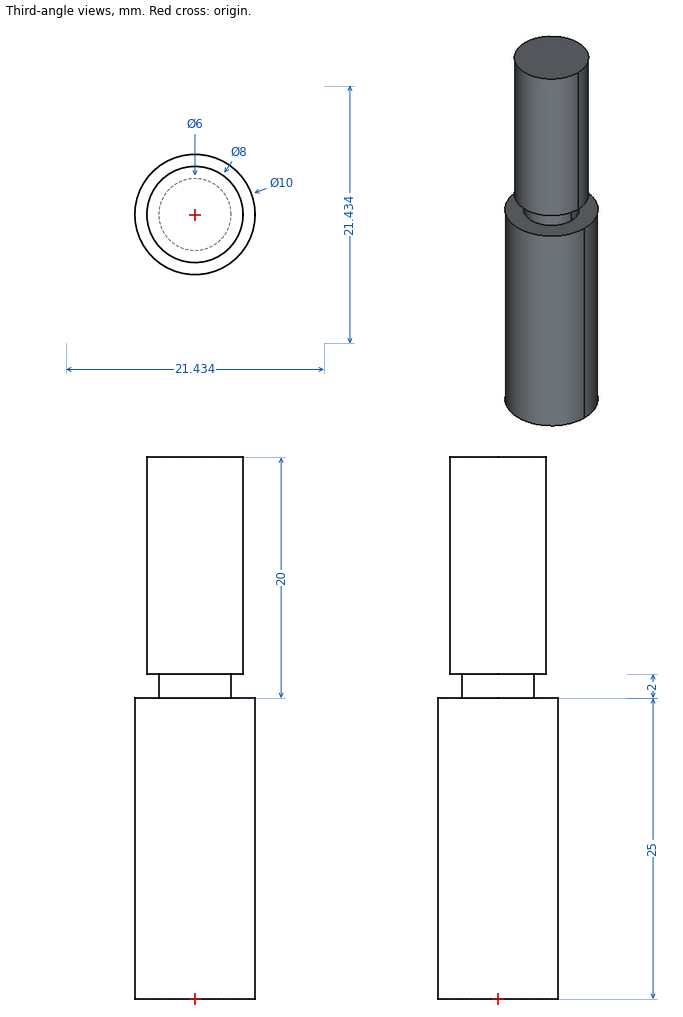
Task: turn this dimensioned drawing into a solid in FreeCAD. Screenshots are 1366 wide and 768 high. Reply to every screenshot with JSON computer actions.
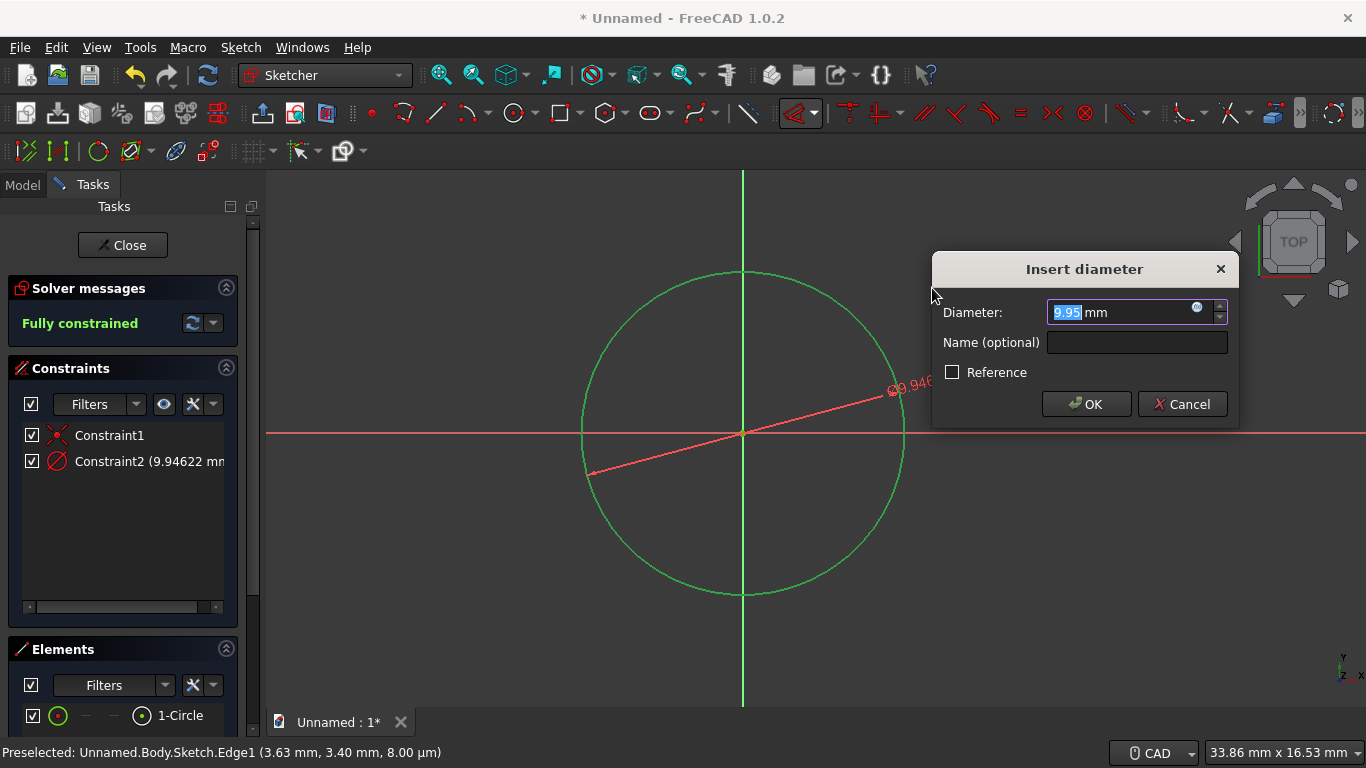
{"action": "type", "text": "10"}
{"action": "key", "text": "Return"}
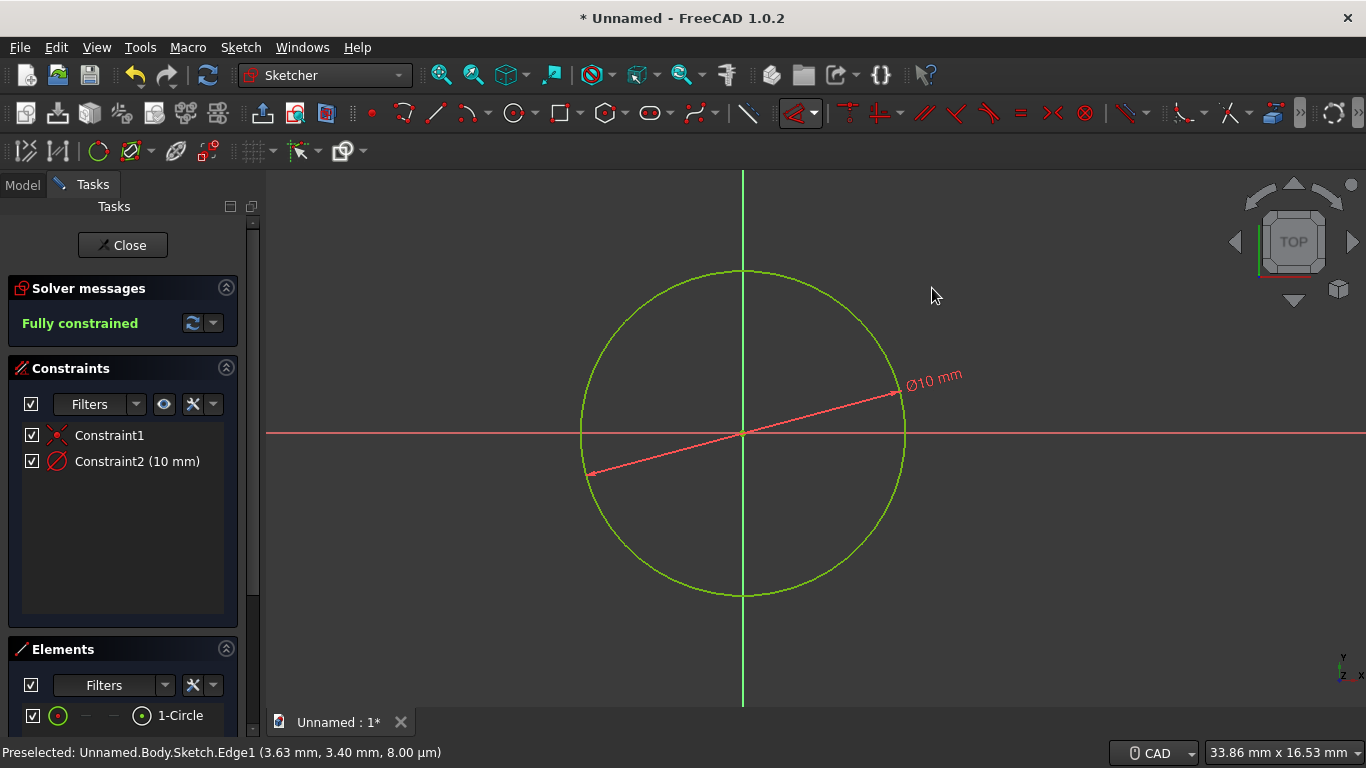
{"action": "left_click", "coordinate": [123, 245]}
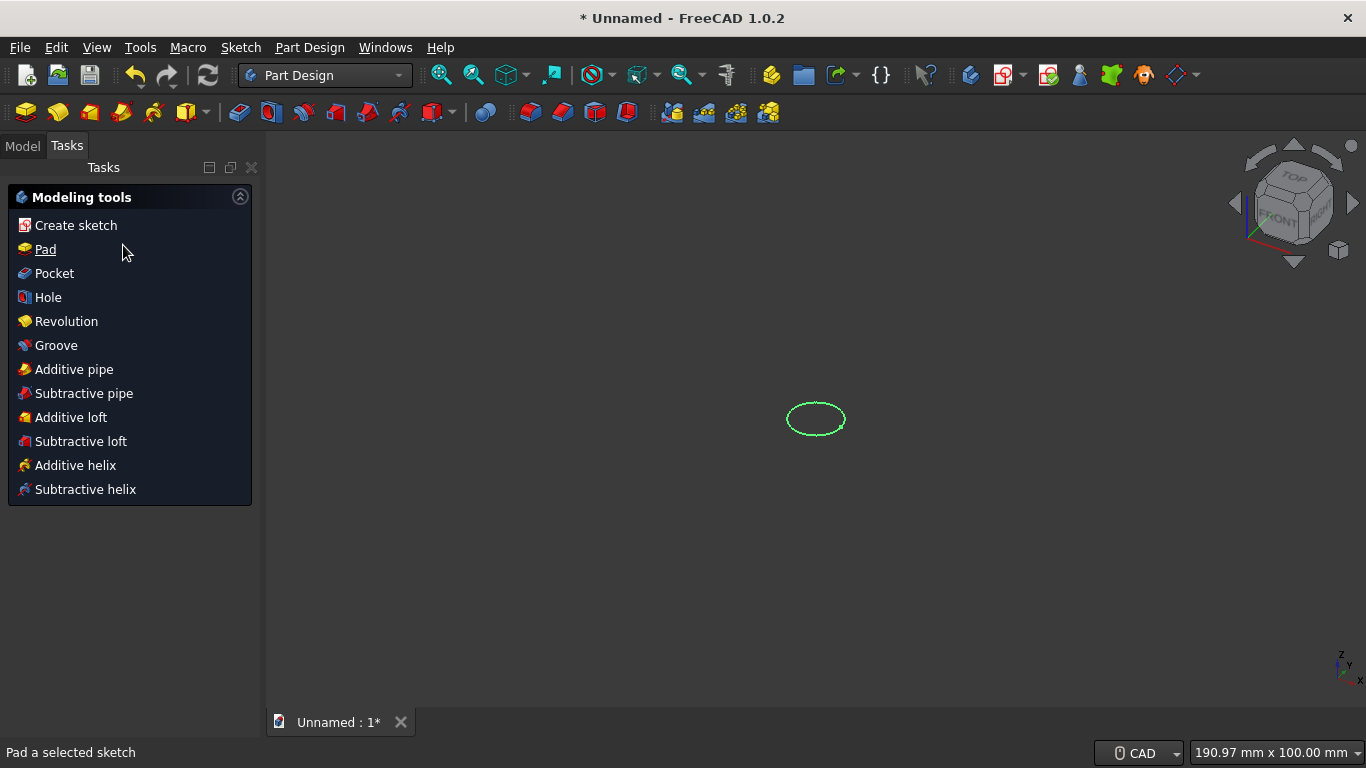
{"action": "left_click", "coordinate": [26, 112]}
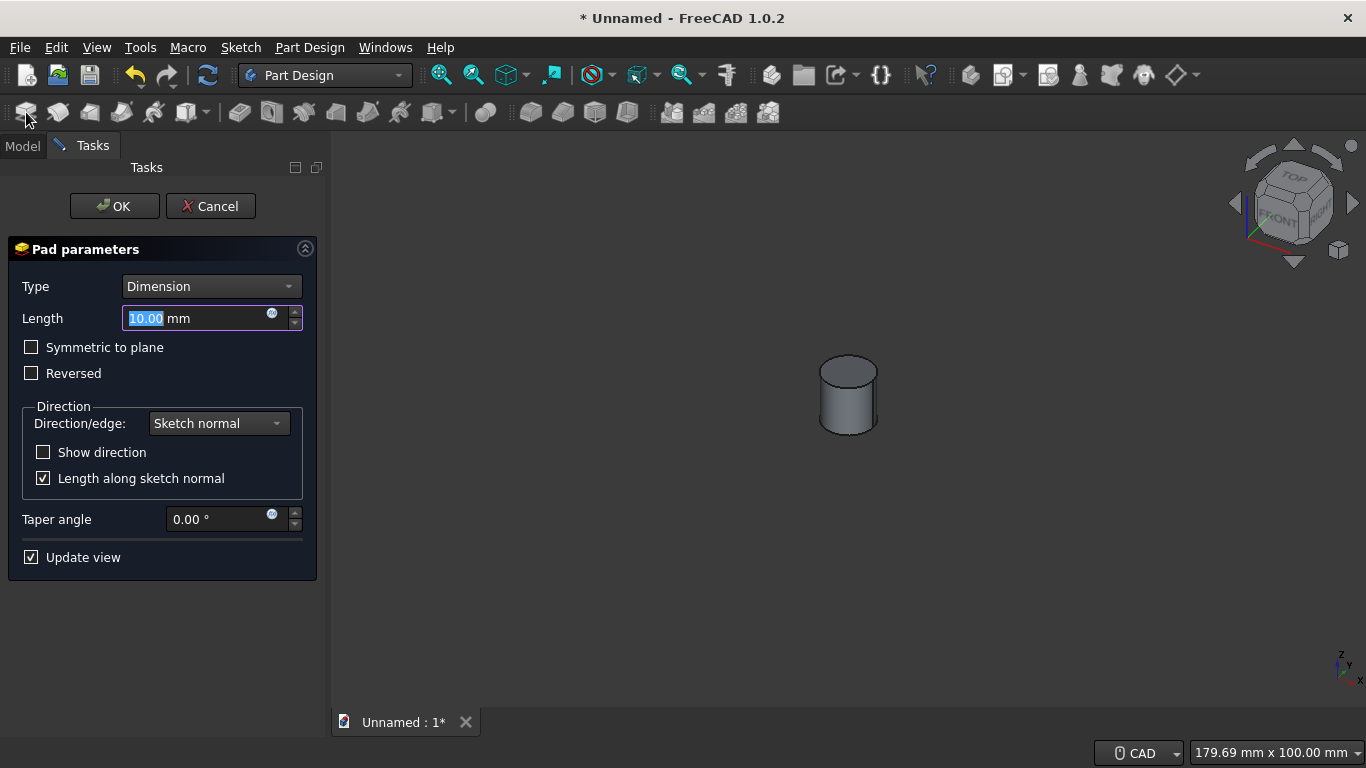
{"action": "type", "text": "25"}
{"action": "key", "text": "Tab"}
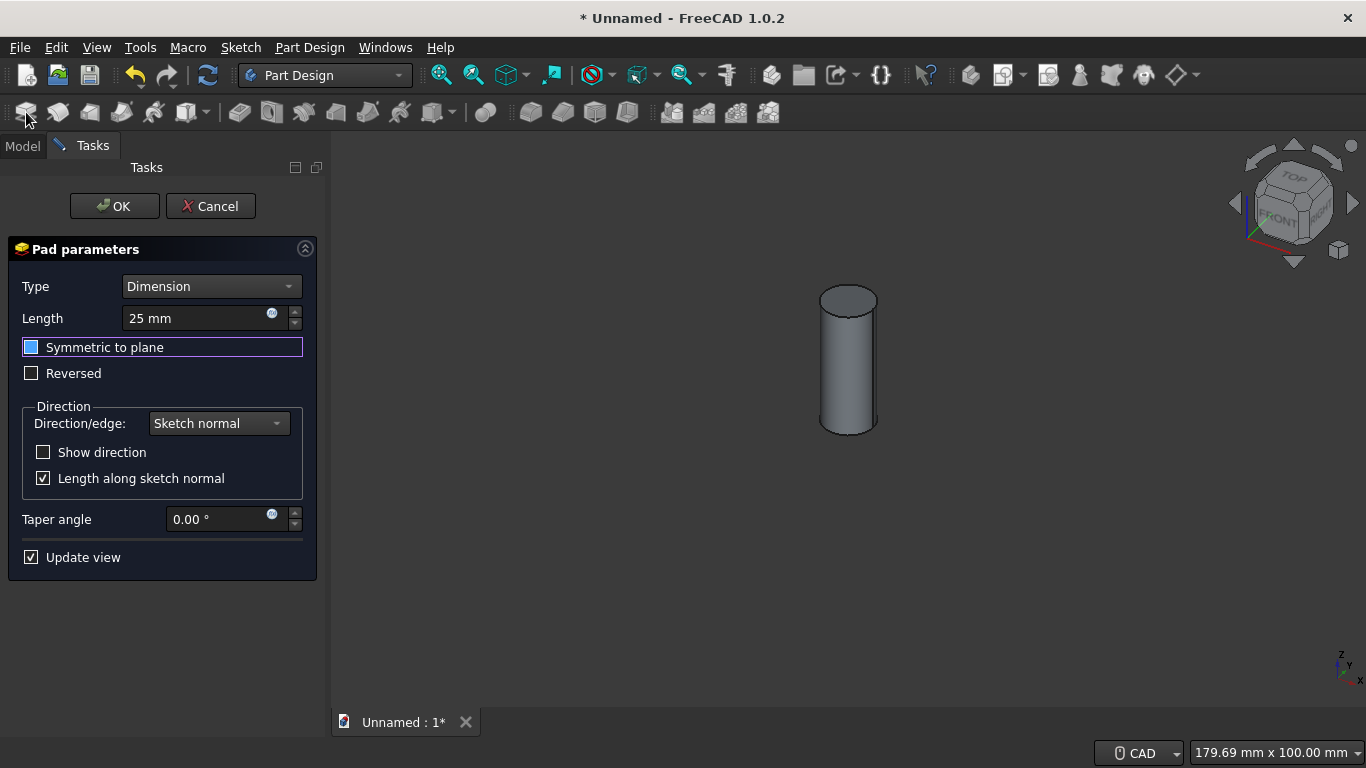
{"action": "left_click", "coordinate": [115, 206]}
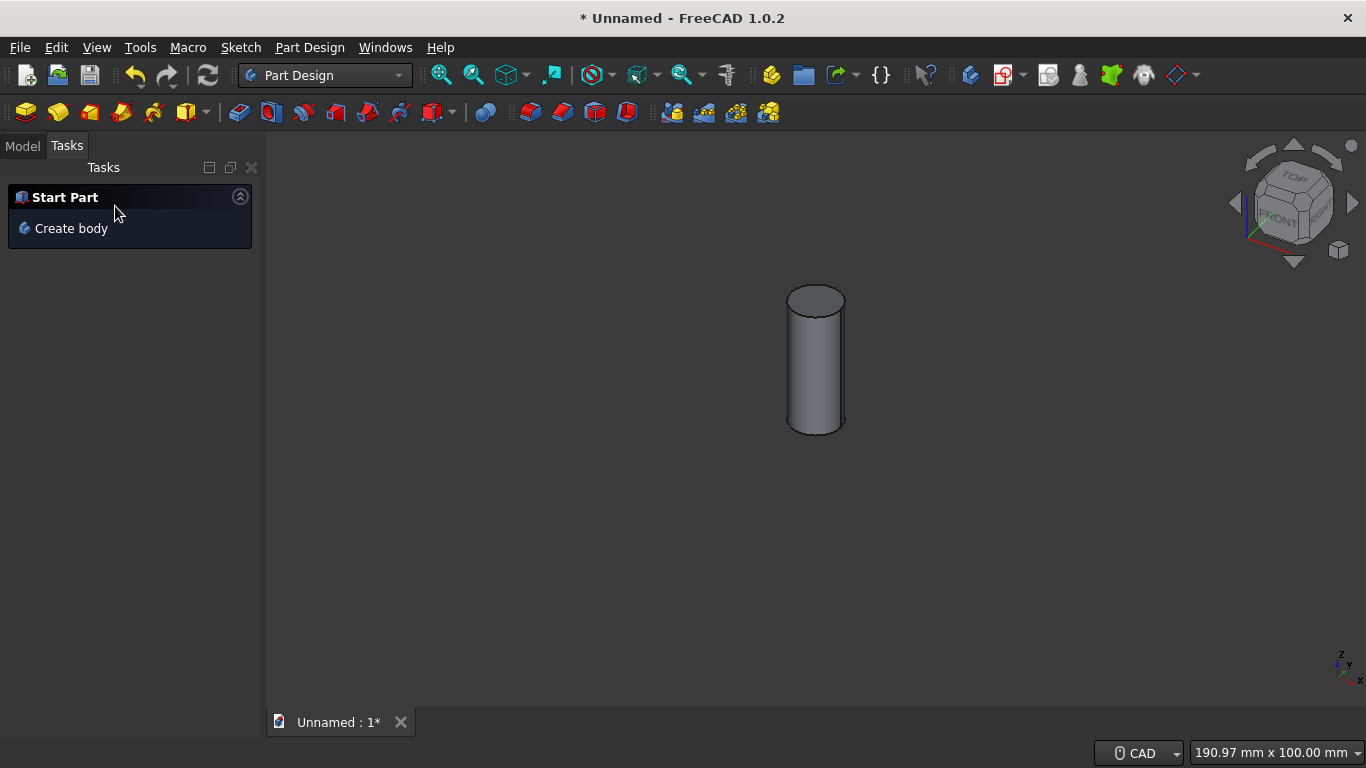
{"action": "left_click", "coordinate": [442, 76]}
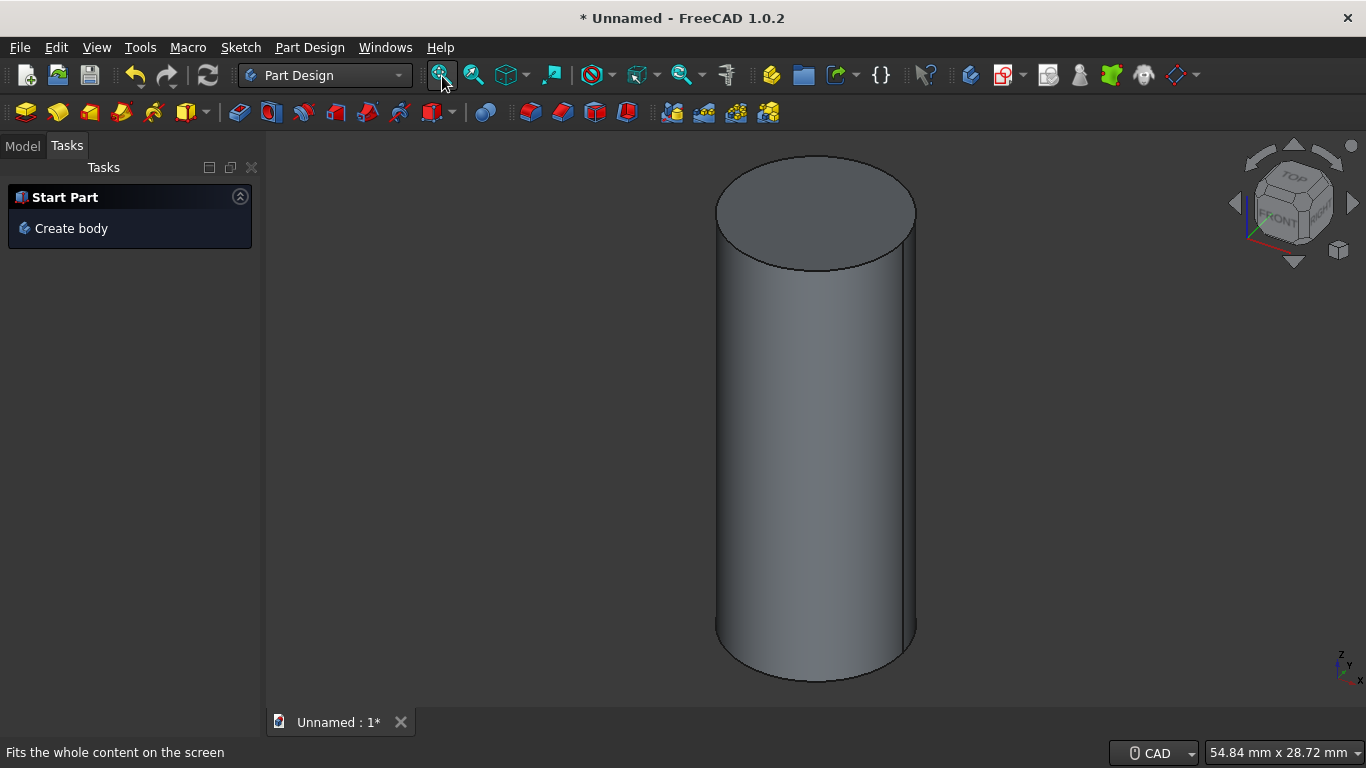
{"action": "left_click", "coordinate": [816, 213]}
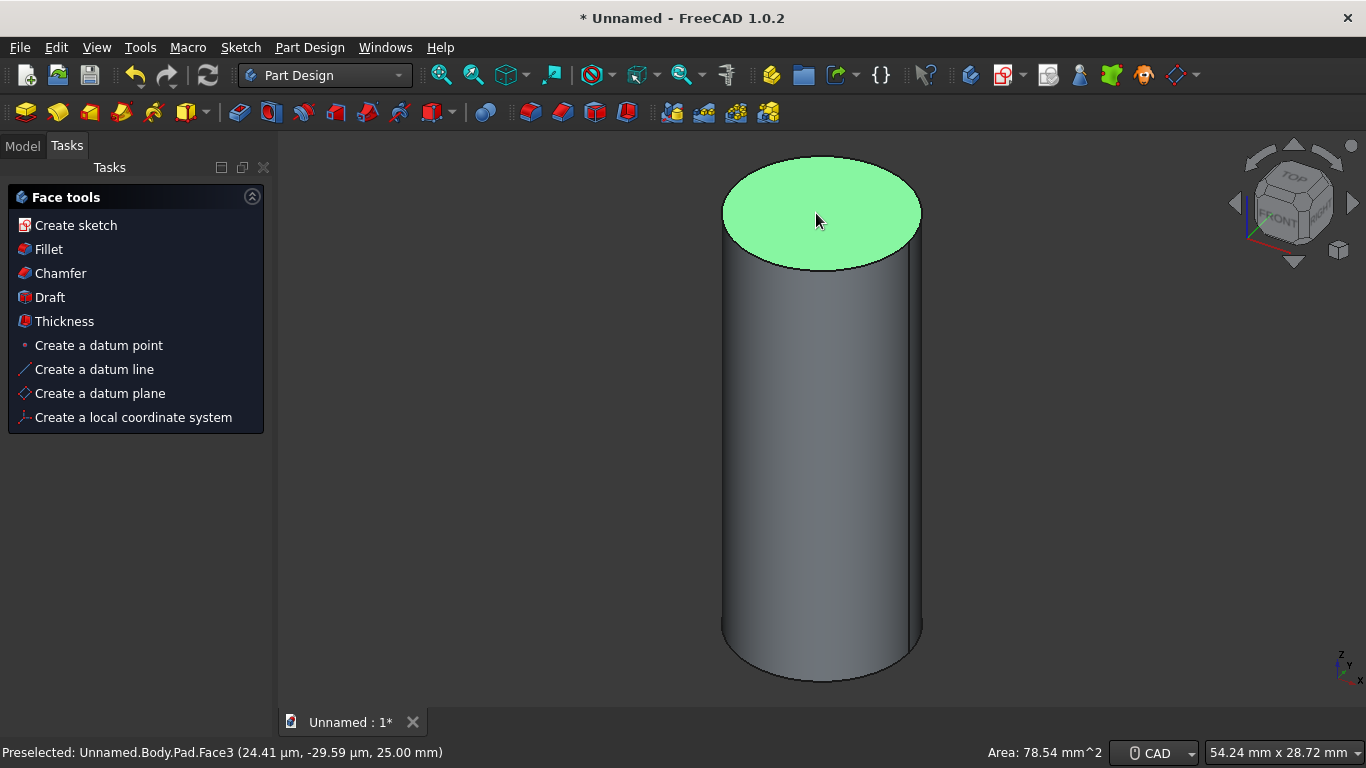
{"action": "left_click", "coordinate": [1004, 76]}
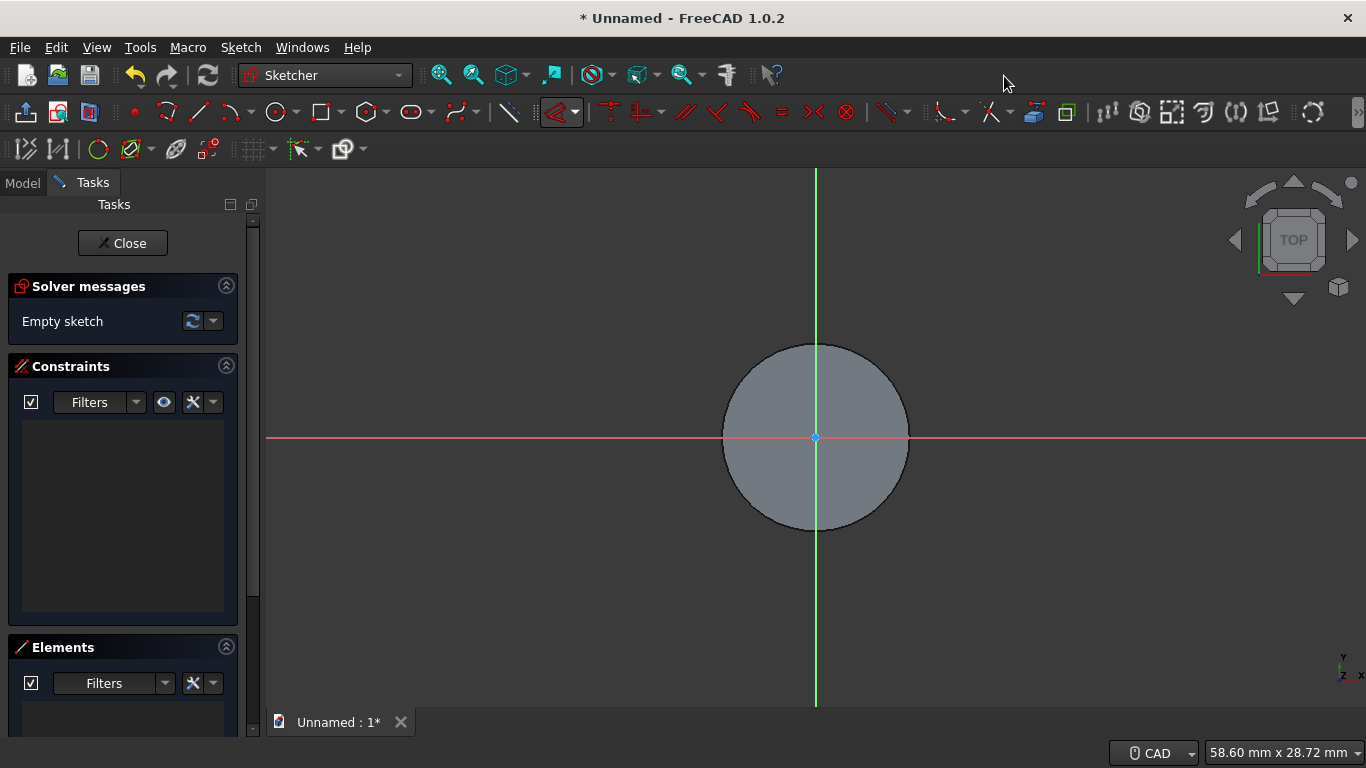
{"action": "scroll", "coordinate": [872, 438], "scroll_direction": "up", "scroll_amount": 4}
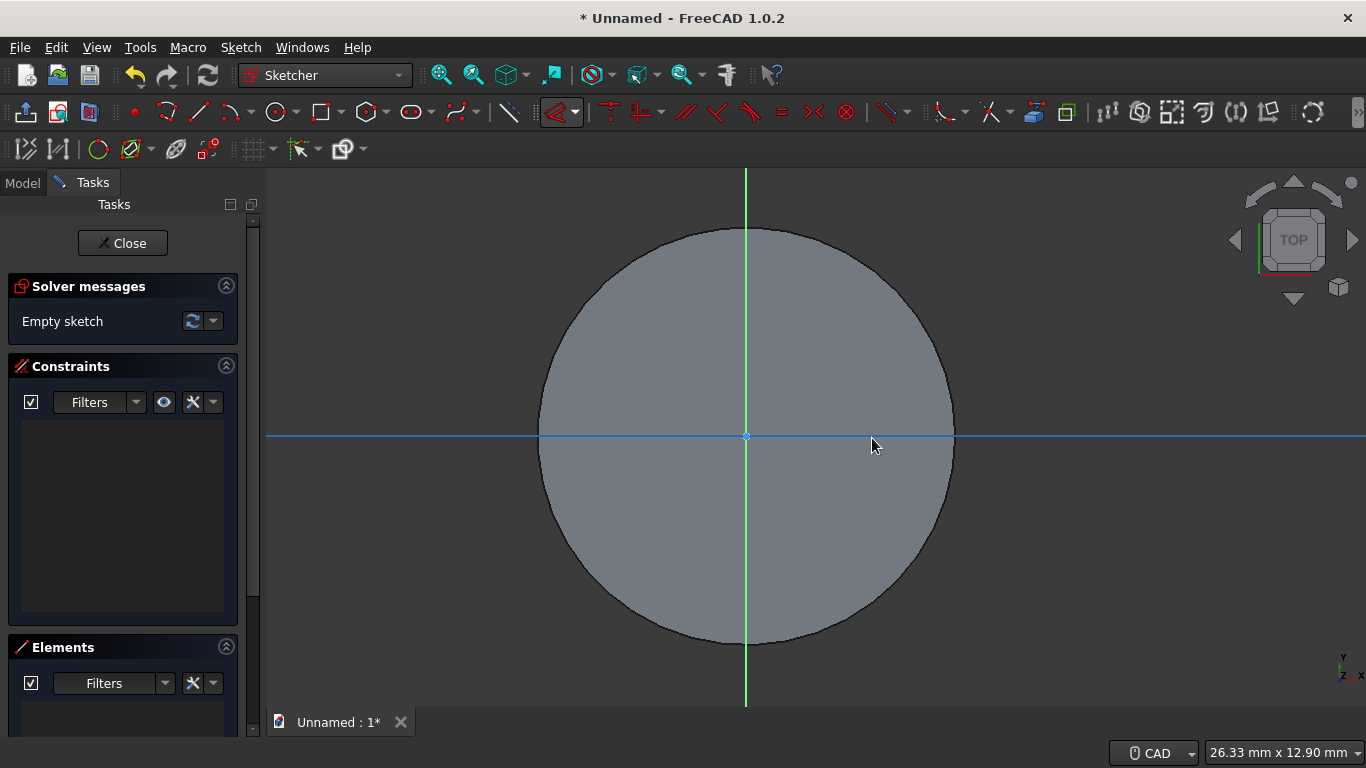
{"action": "key", "text": "g c"}